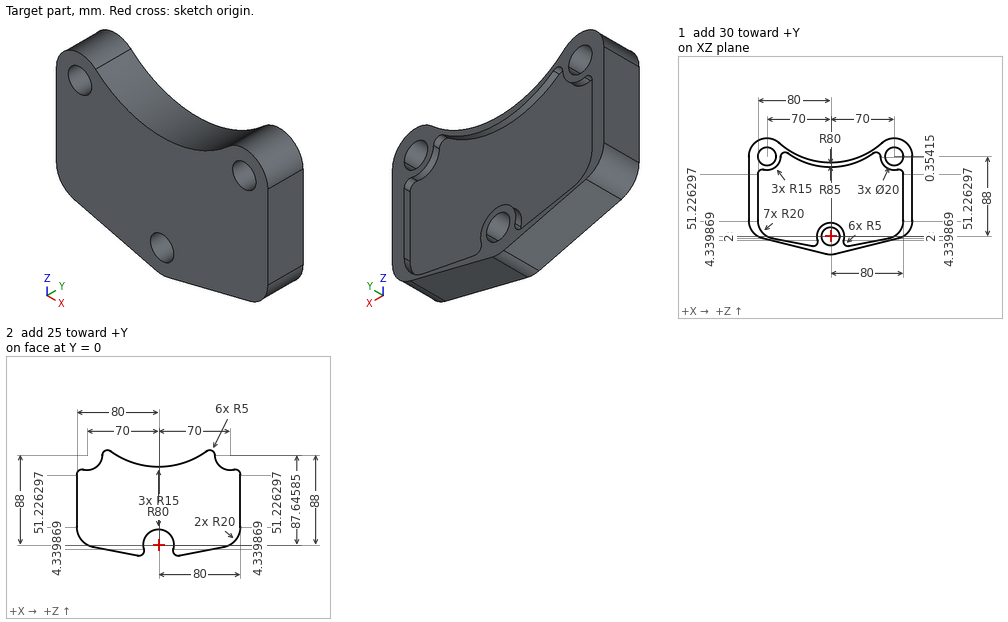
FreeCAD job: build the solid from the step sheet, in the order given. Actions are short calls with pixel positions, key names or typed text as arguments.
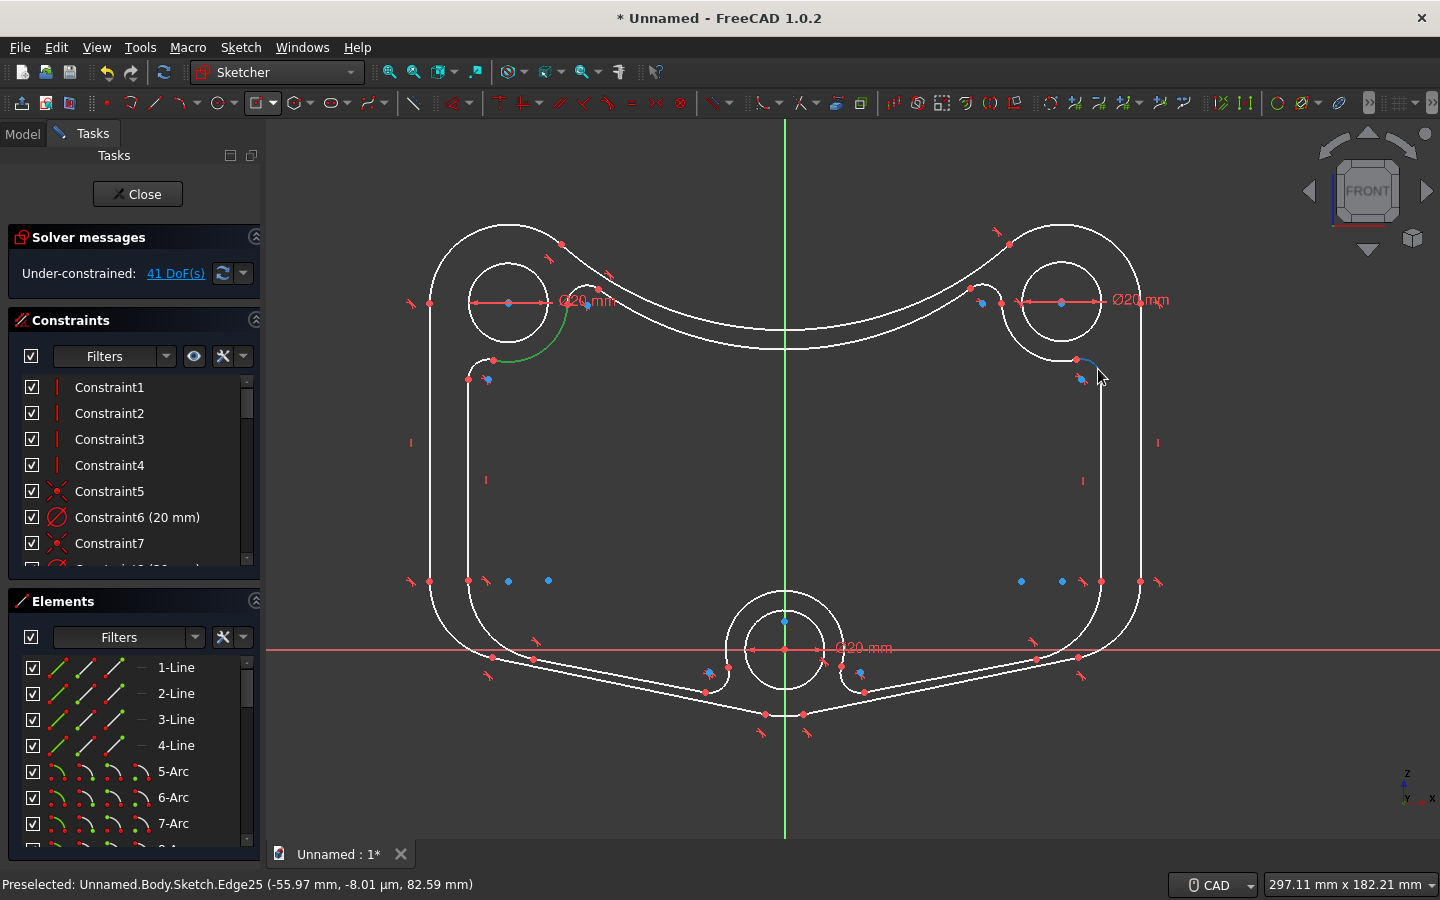
scroll(483, 360, up, 2)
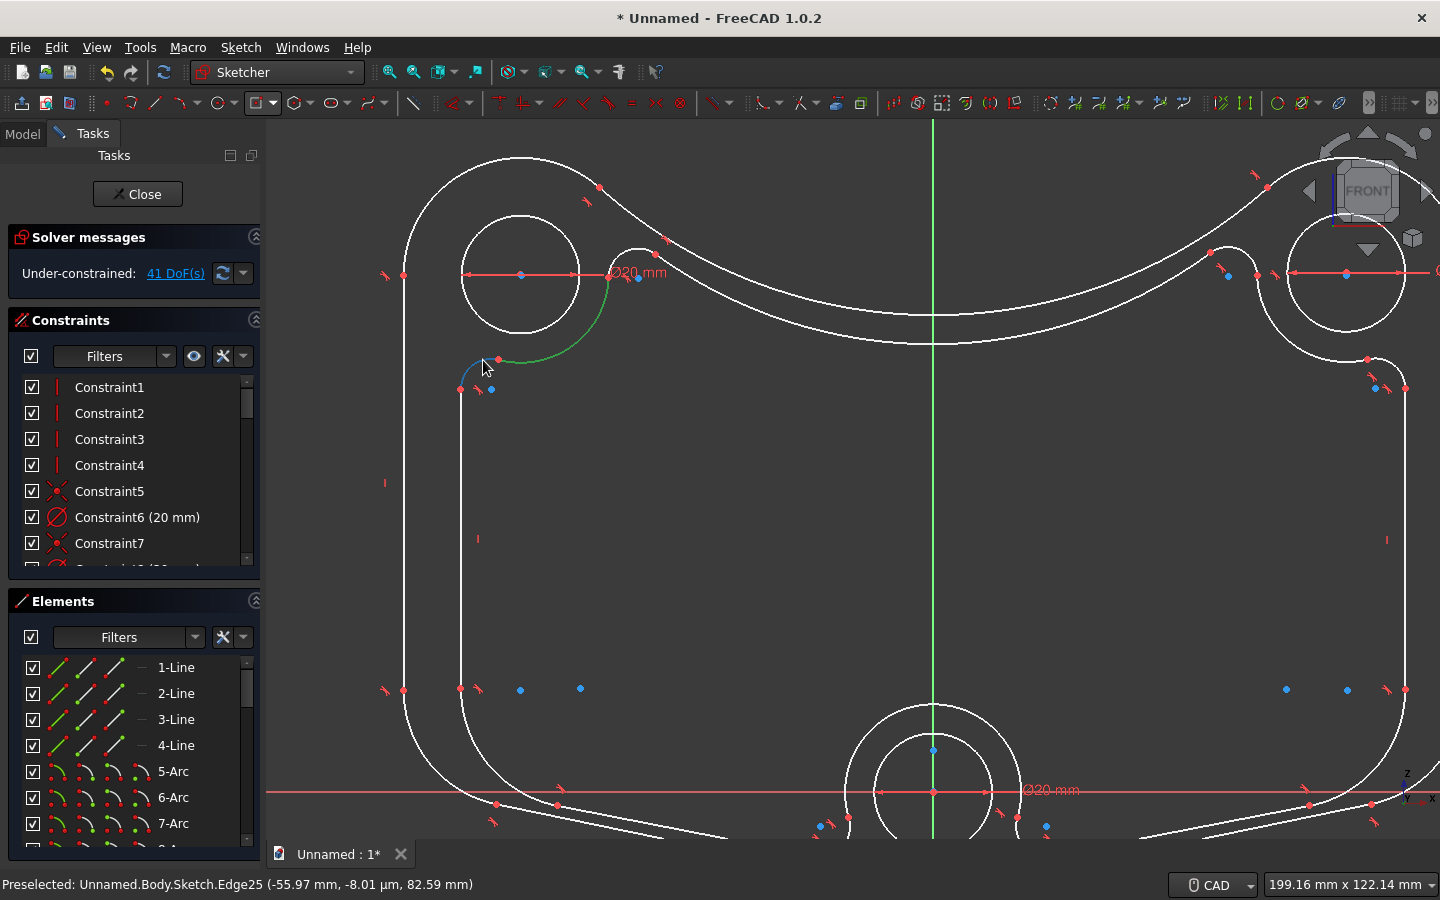
click(482, 360)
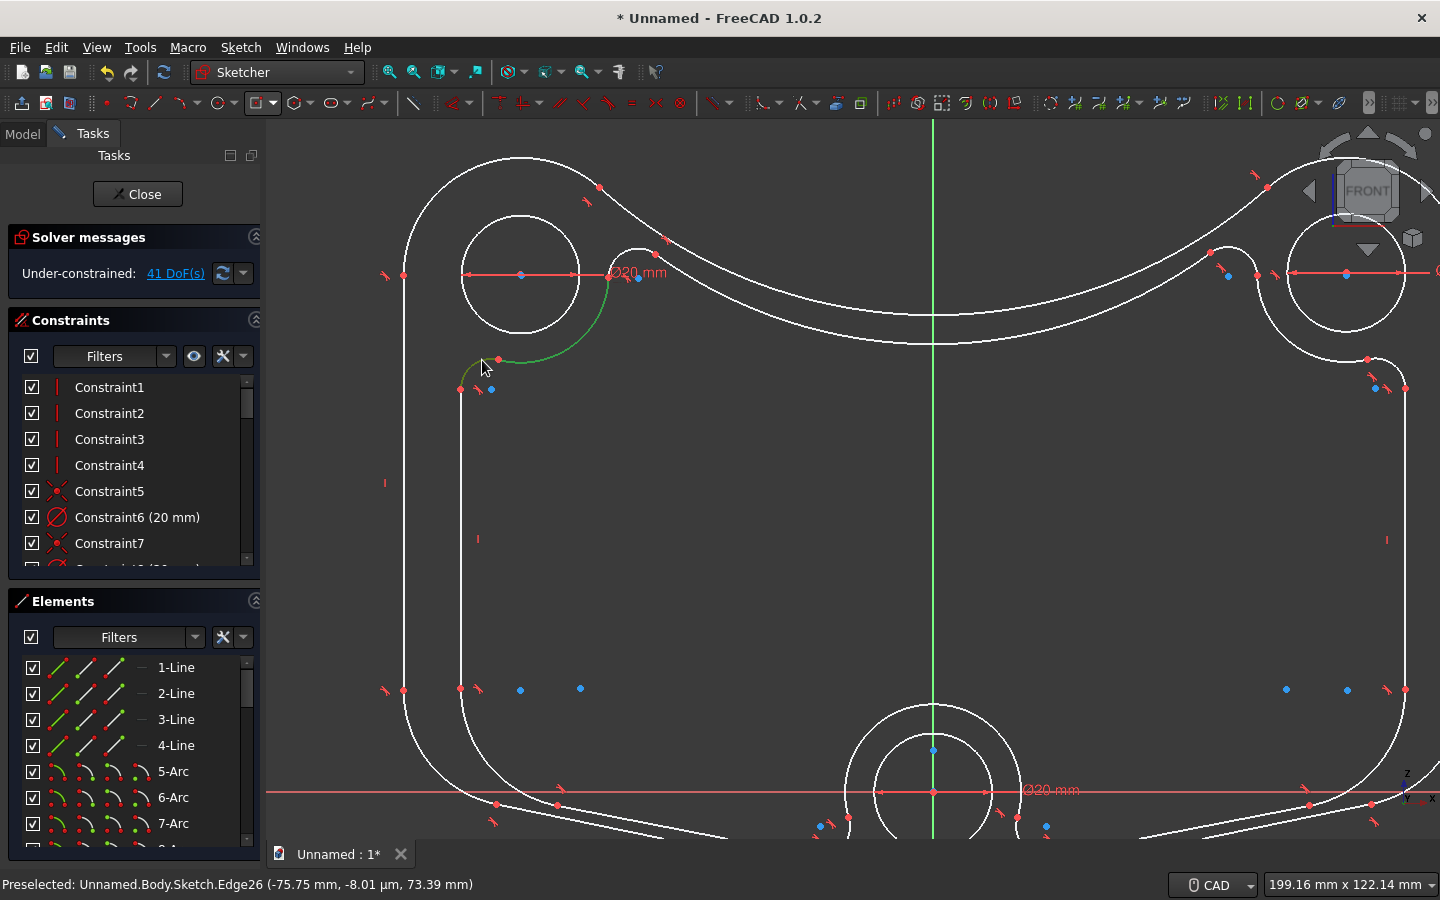
click(608, 104)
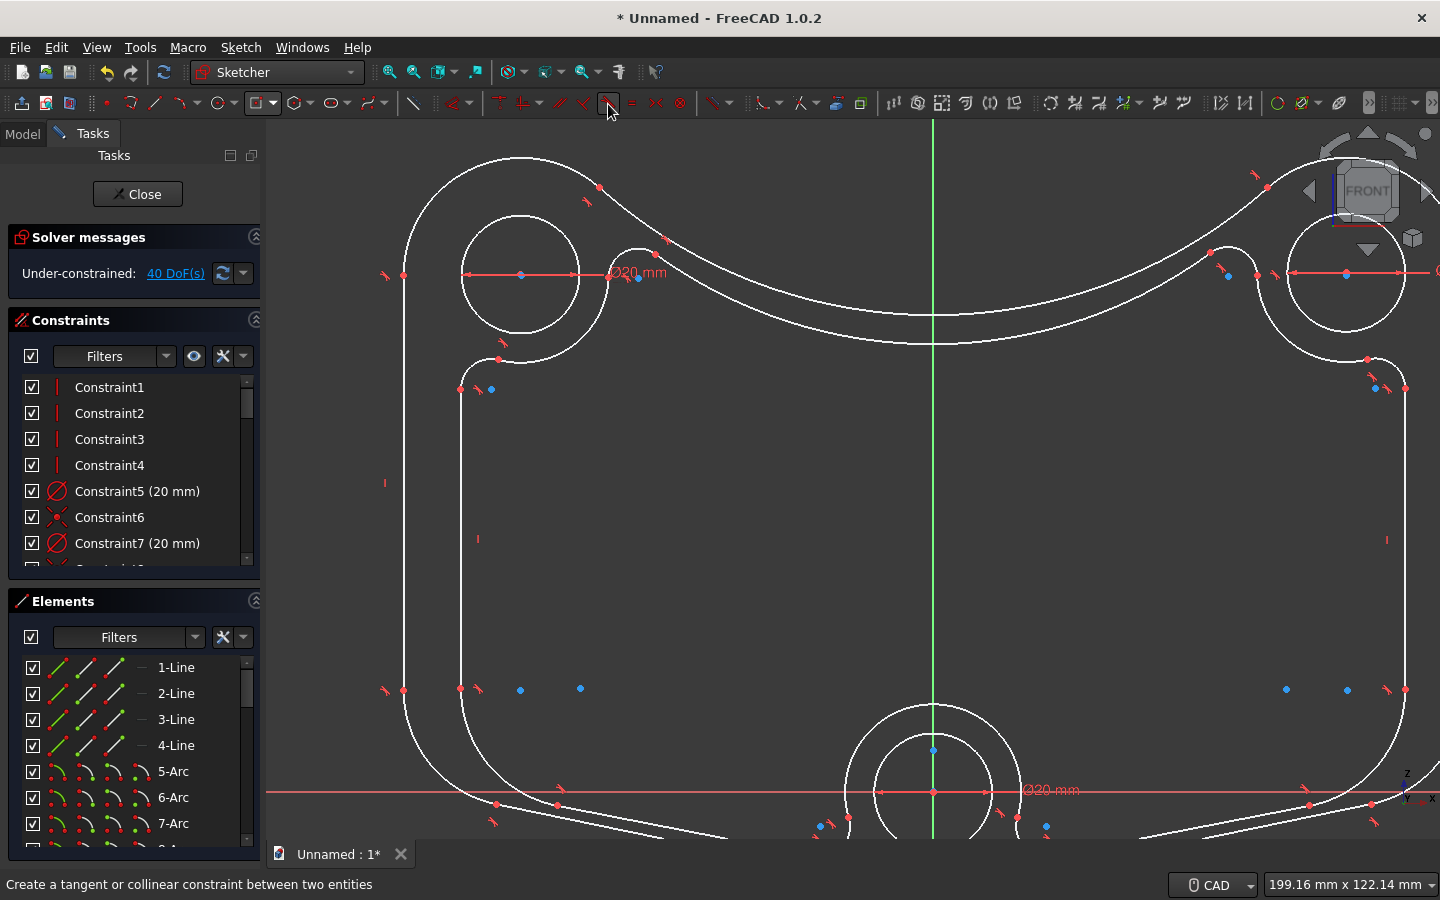
click(562, 233)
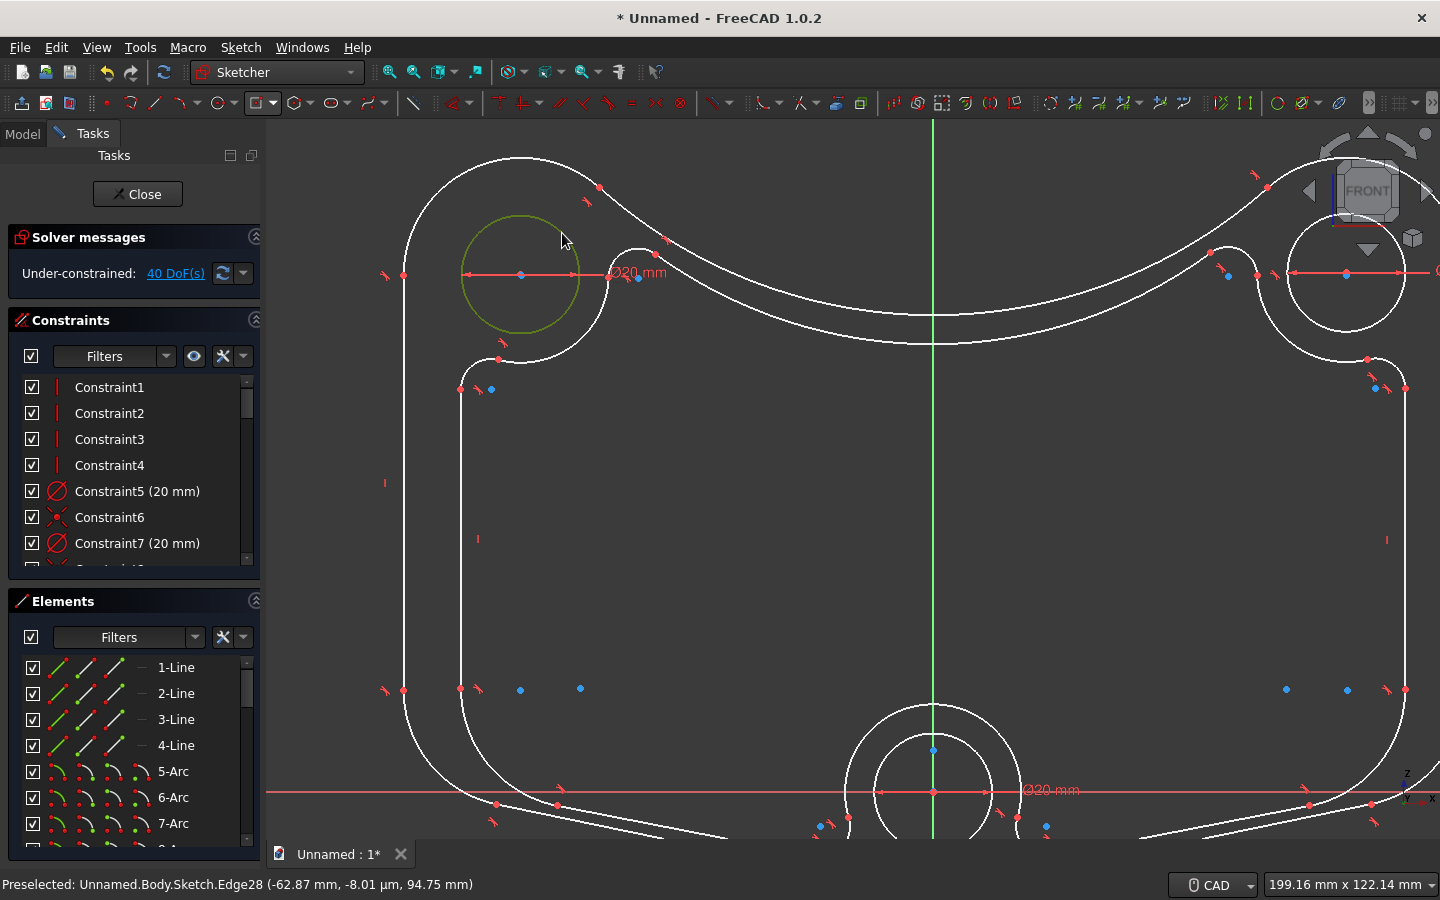
click(526, 158)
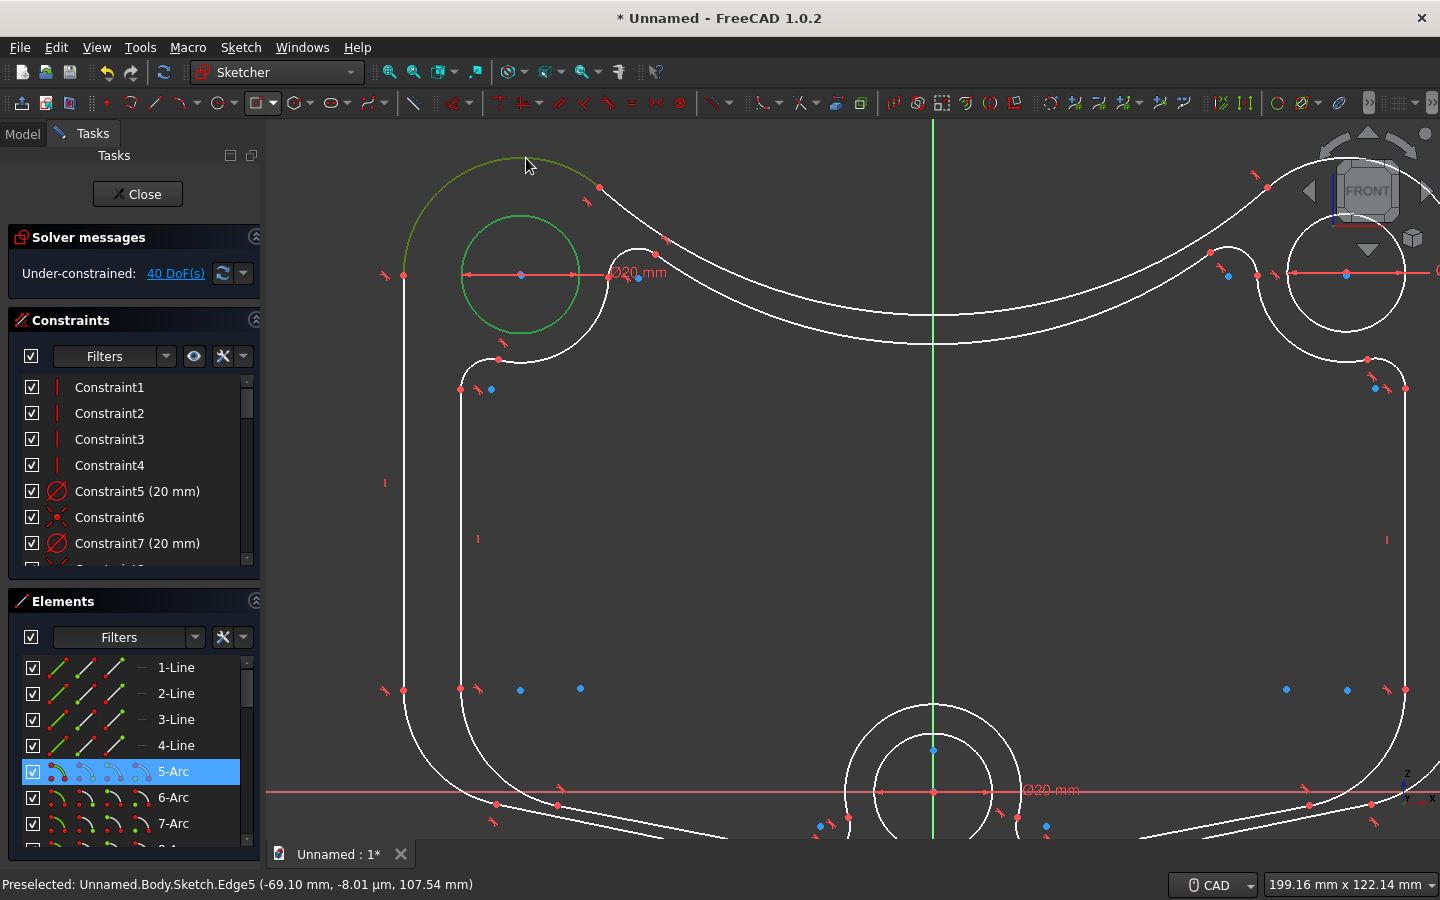
click(500, 104)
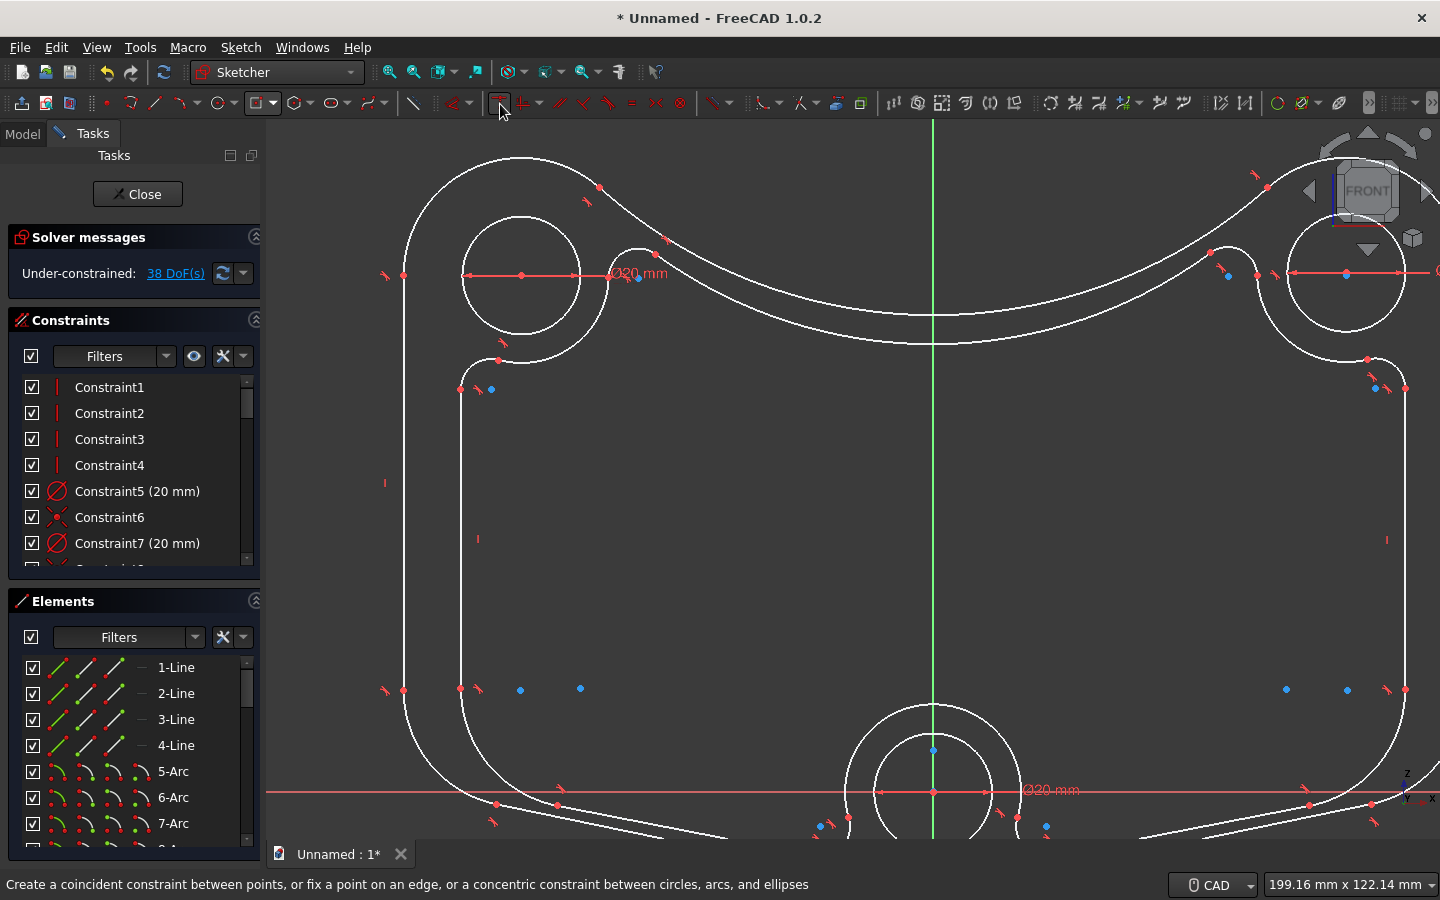
scroll(482, 360, down, 2)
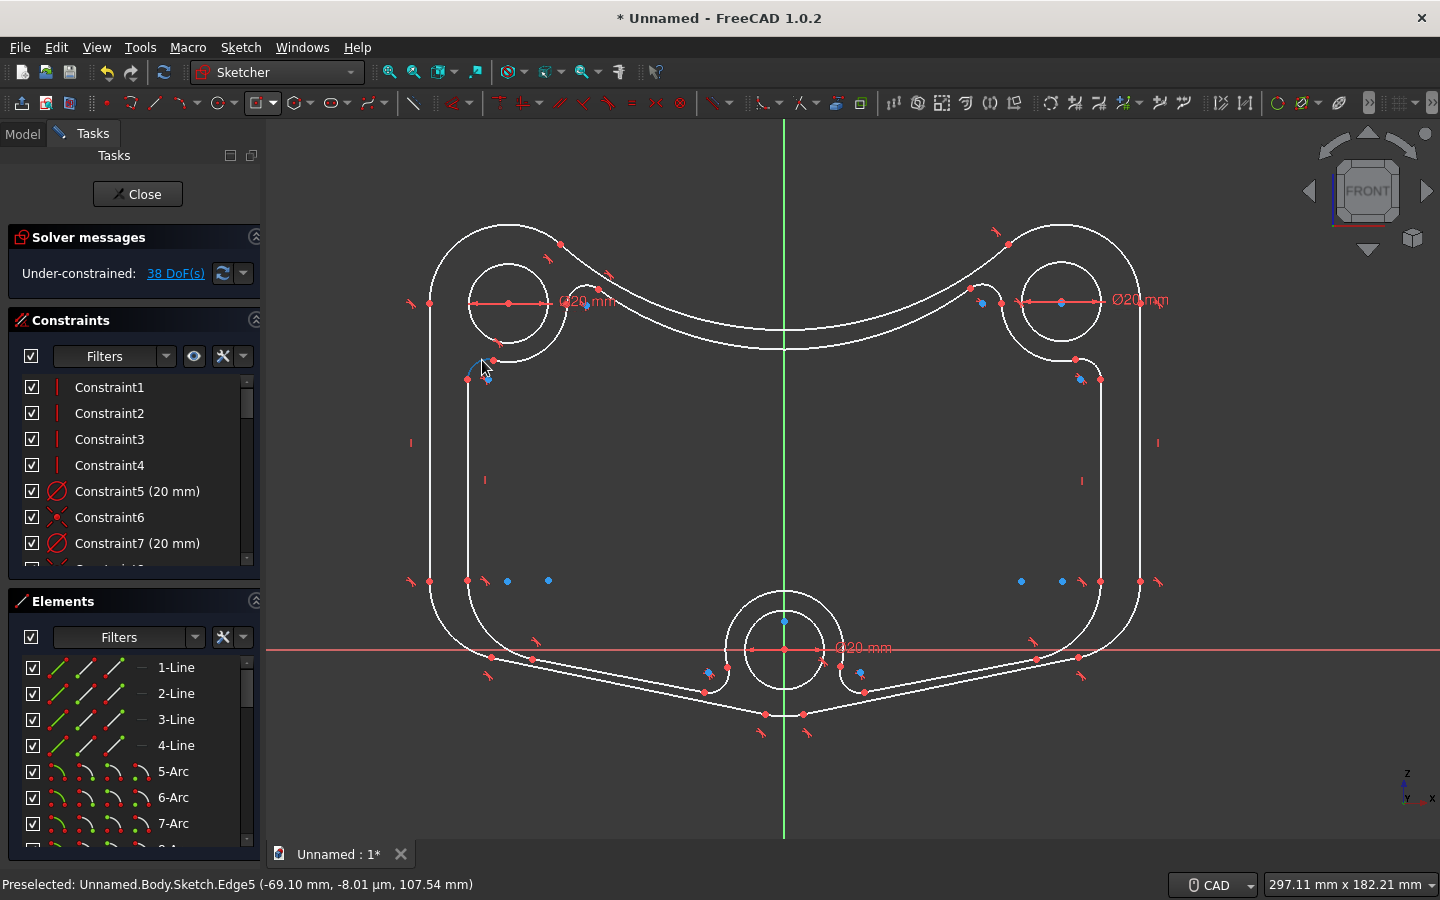
click(1089, 274)